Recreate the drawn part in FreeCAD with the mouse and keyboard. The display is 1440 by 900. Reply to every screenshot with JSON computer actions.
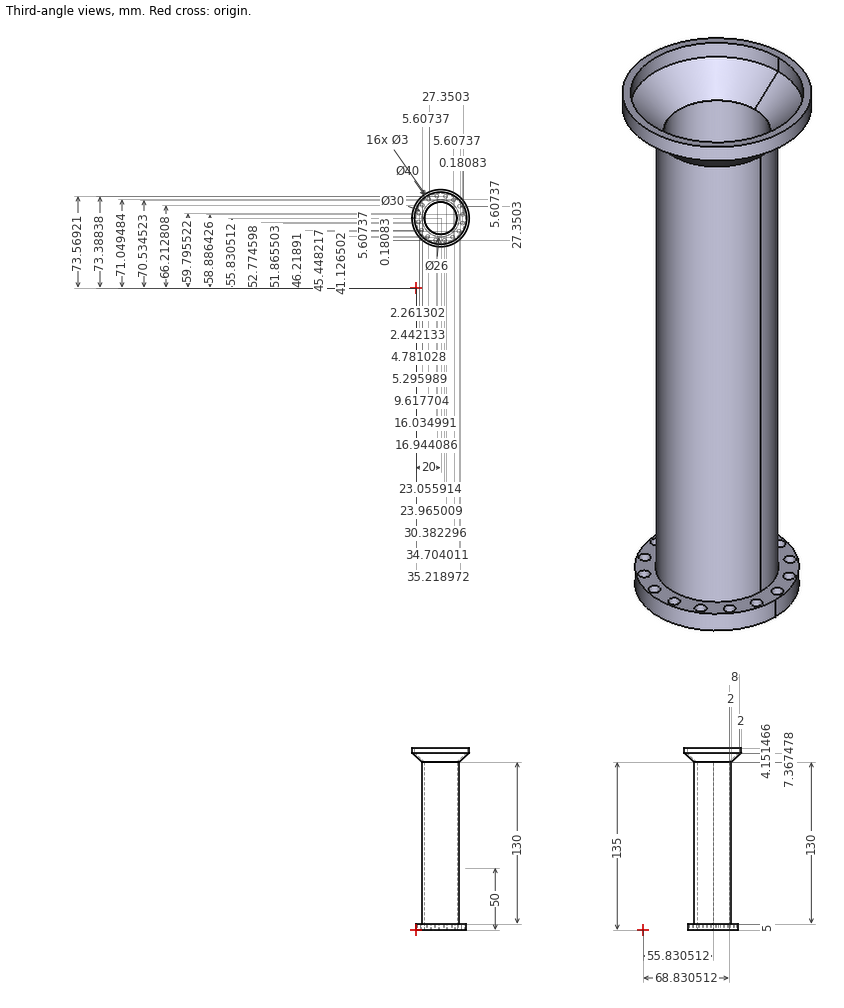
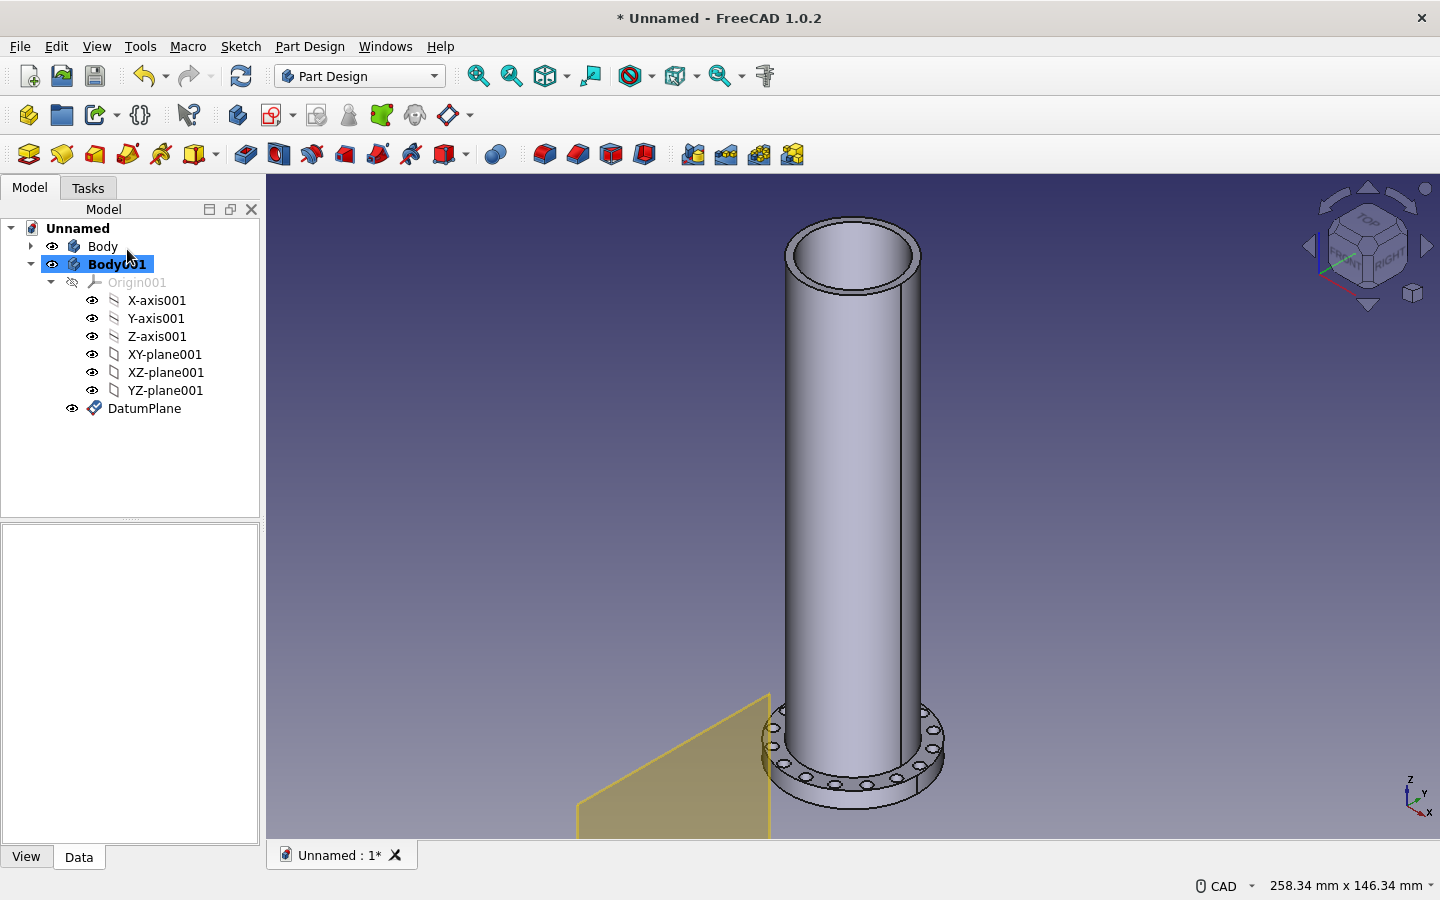
{"action": "left_click", "coordinate": [117, 408]}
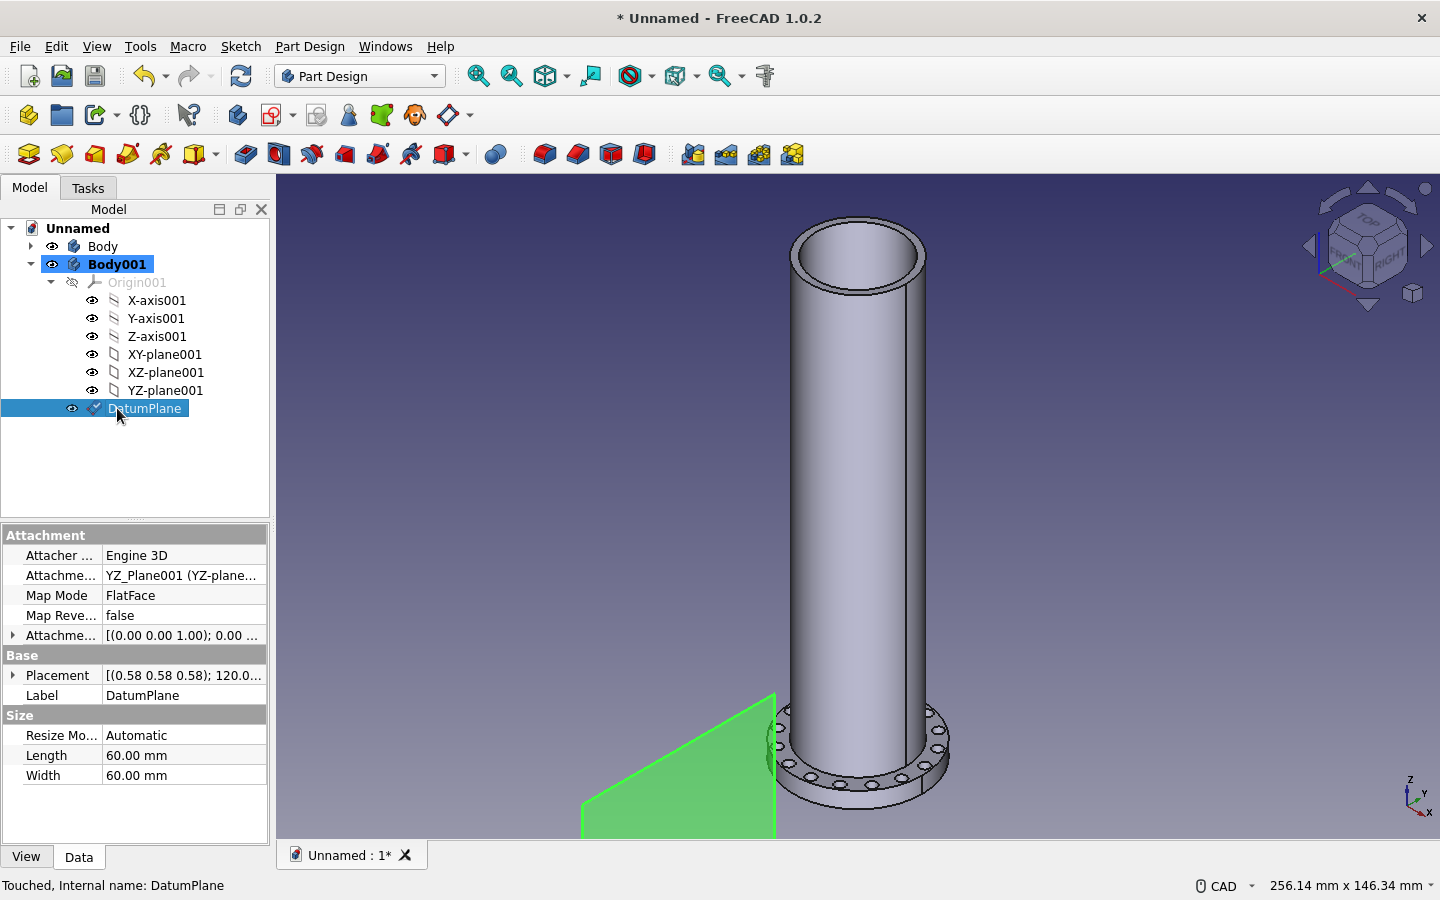
{"action": "left_click", "coordinate": [270, 116]}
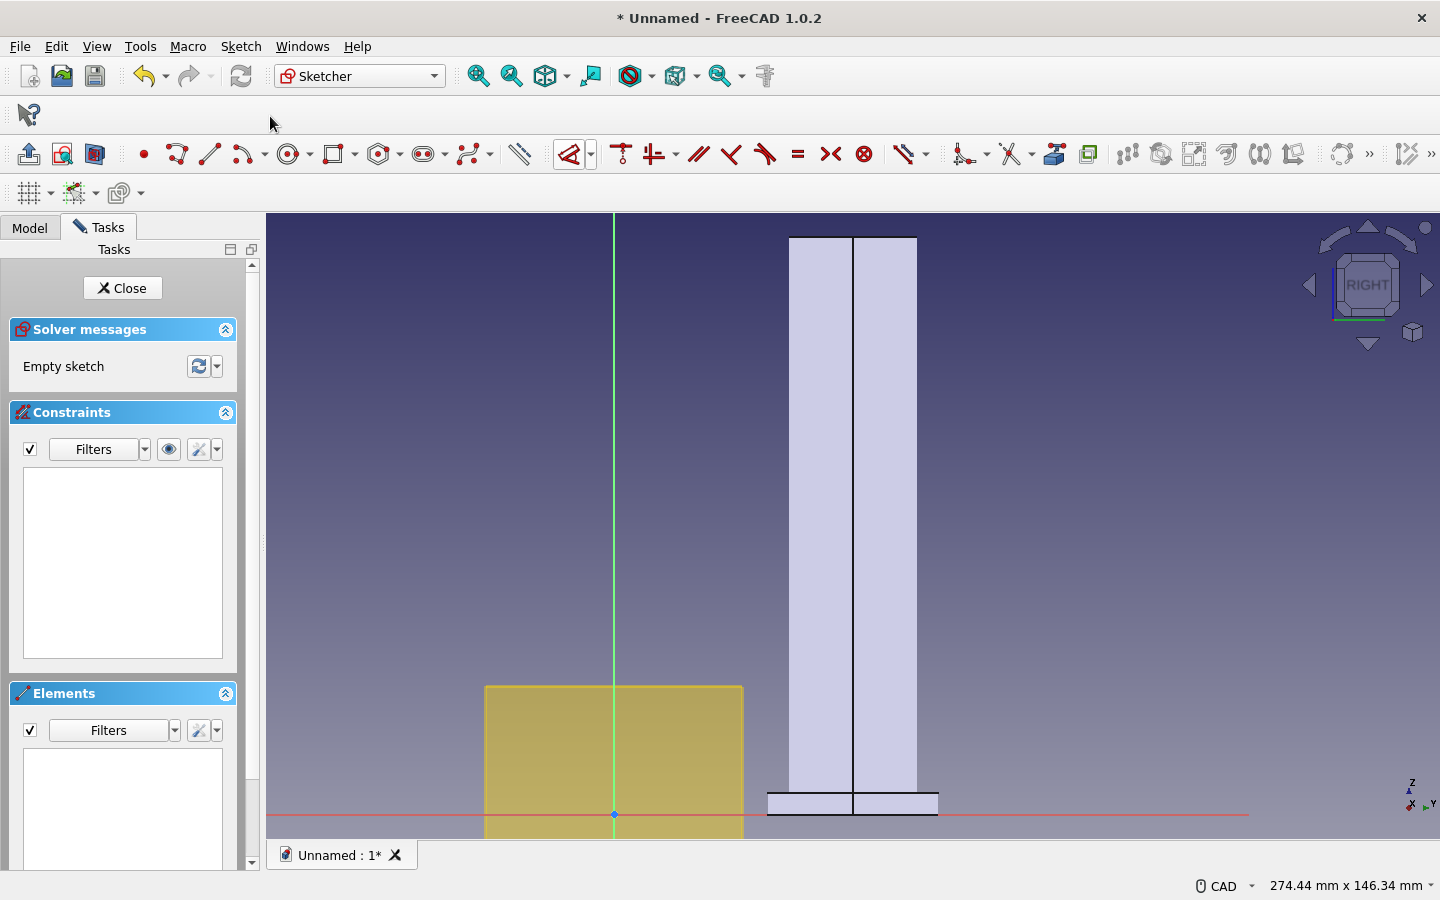
{"action": "scroll", "coordinate": [784, 526], "scroll_direction": "down", "scroll_amount": 5}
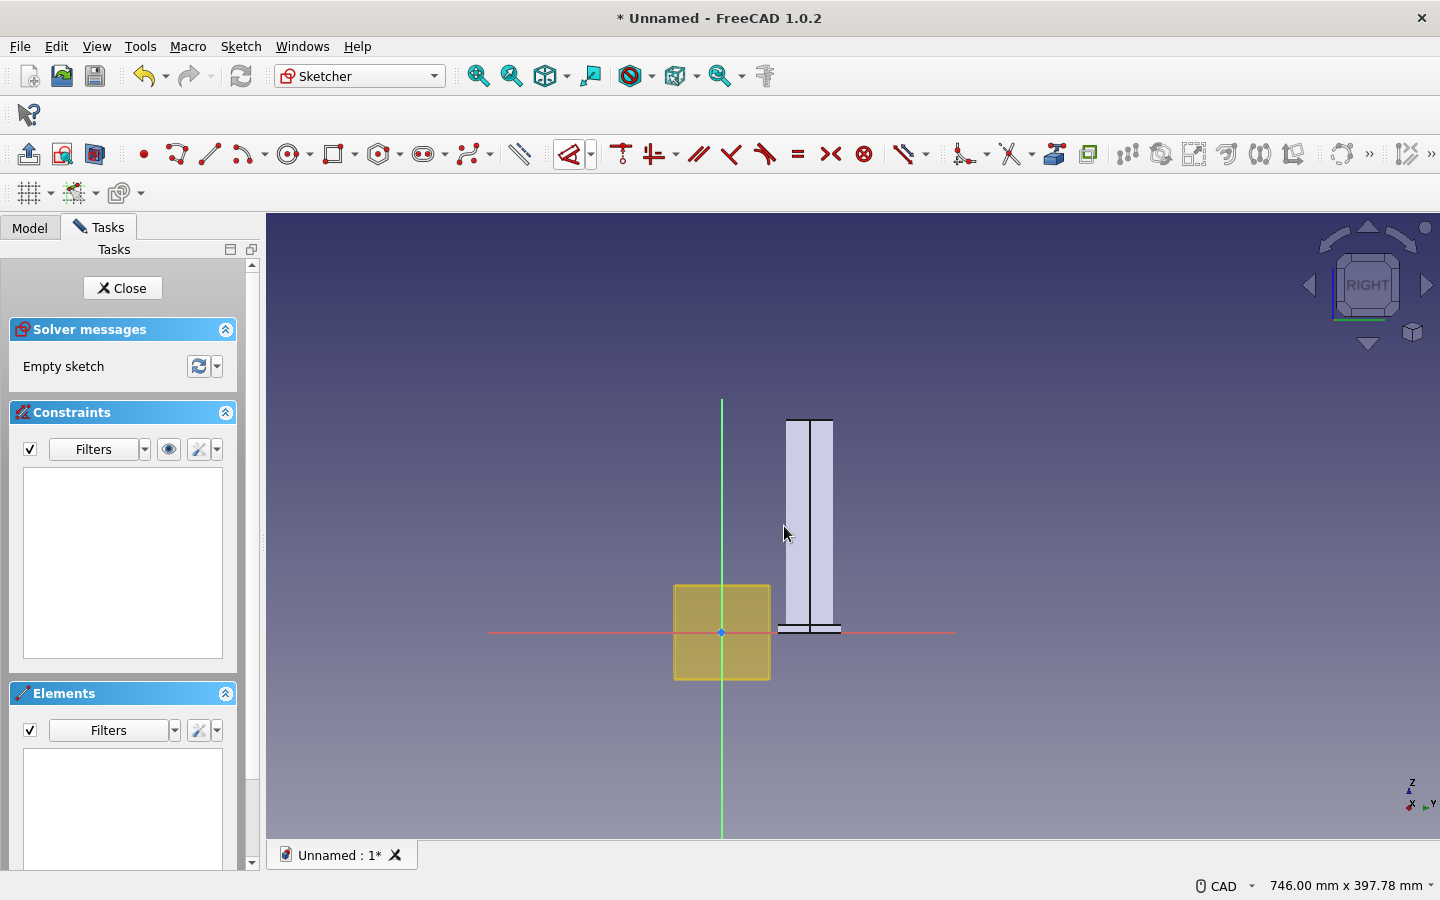
{"action": "scroll", "coordinate": [830, 405], "scroll_direction": "up", "scroll_amount": 15}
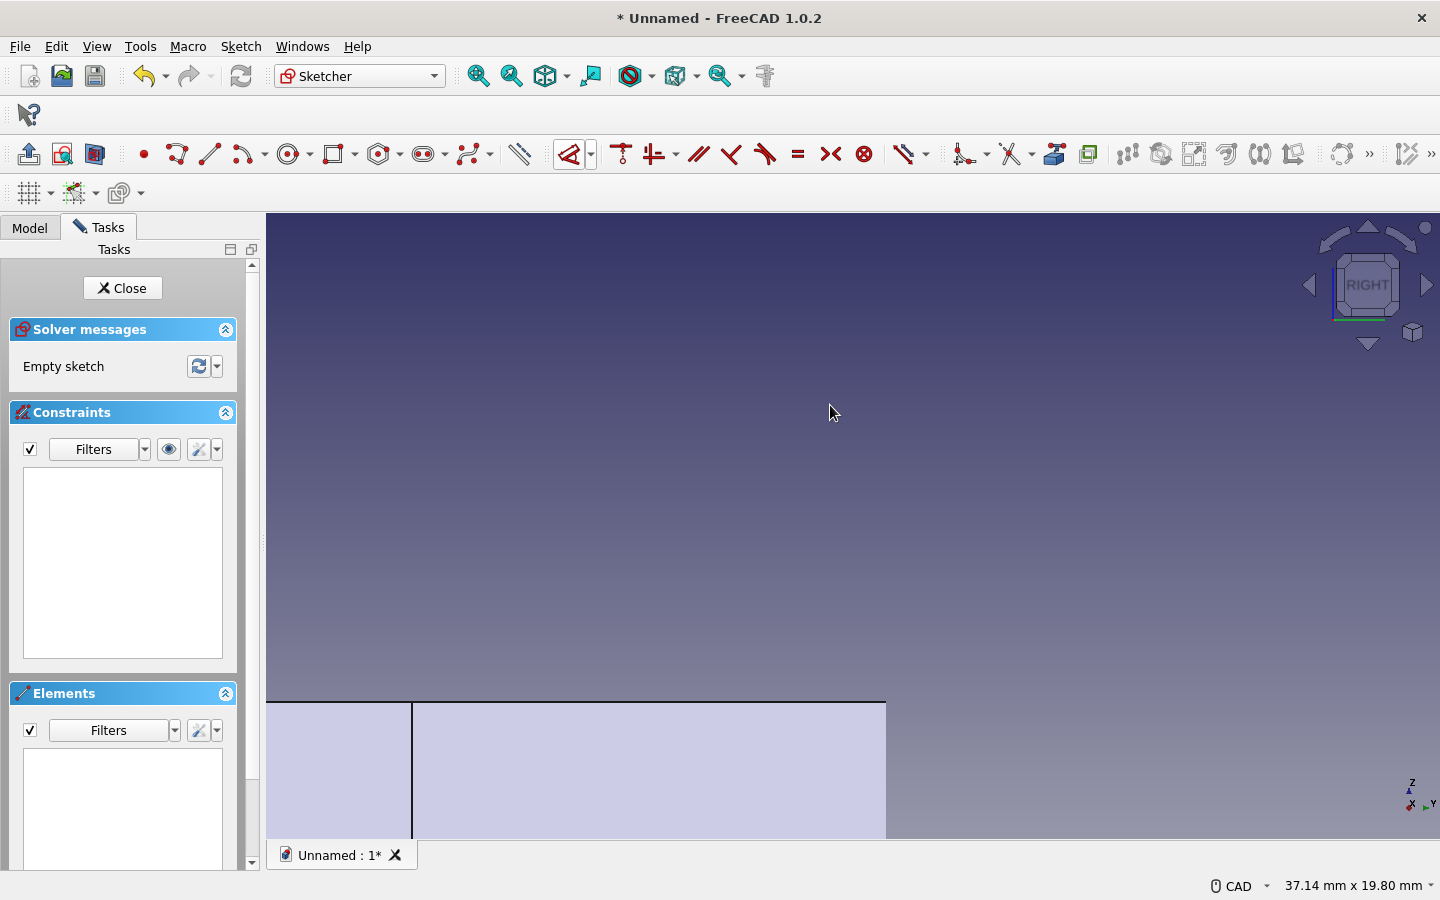
{"action": "left_click", "coordinate": [177, 154]}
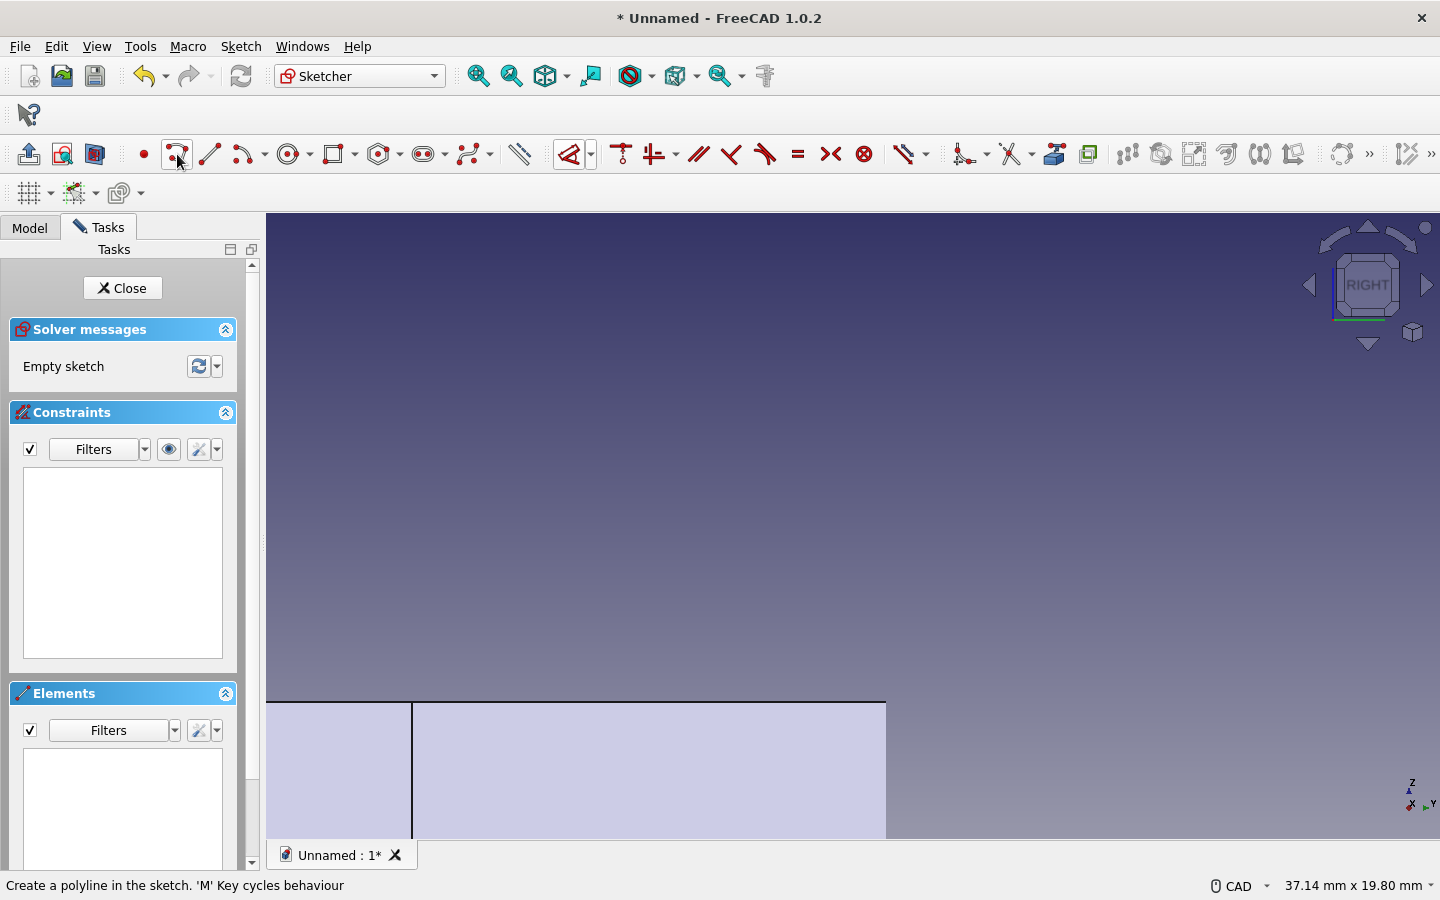
{"action": "left_click", "coordinate": [823, 702]}
{"action": "left_click", "coordinate": [1076, 469]}
{"action": "left_click", "coordinate": [1076, 338]}
{"action": "left_click", "coordinate": [1139, 338]}
{"action": "left_click", "coordinate": [1139, 469]}
{"action": "left_click", "coordinate": [886, 702]}
{"action": "left_click", "coordinate": [823, 703]}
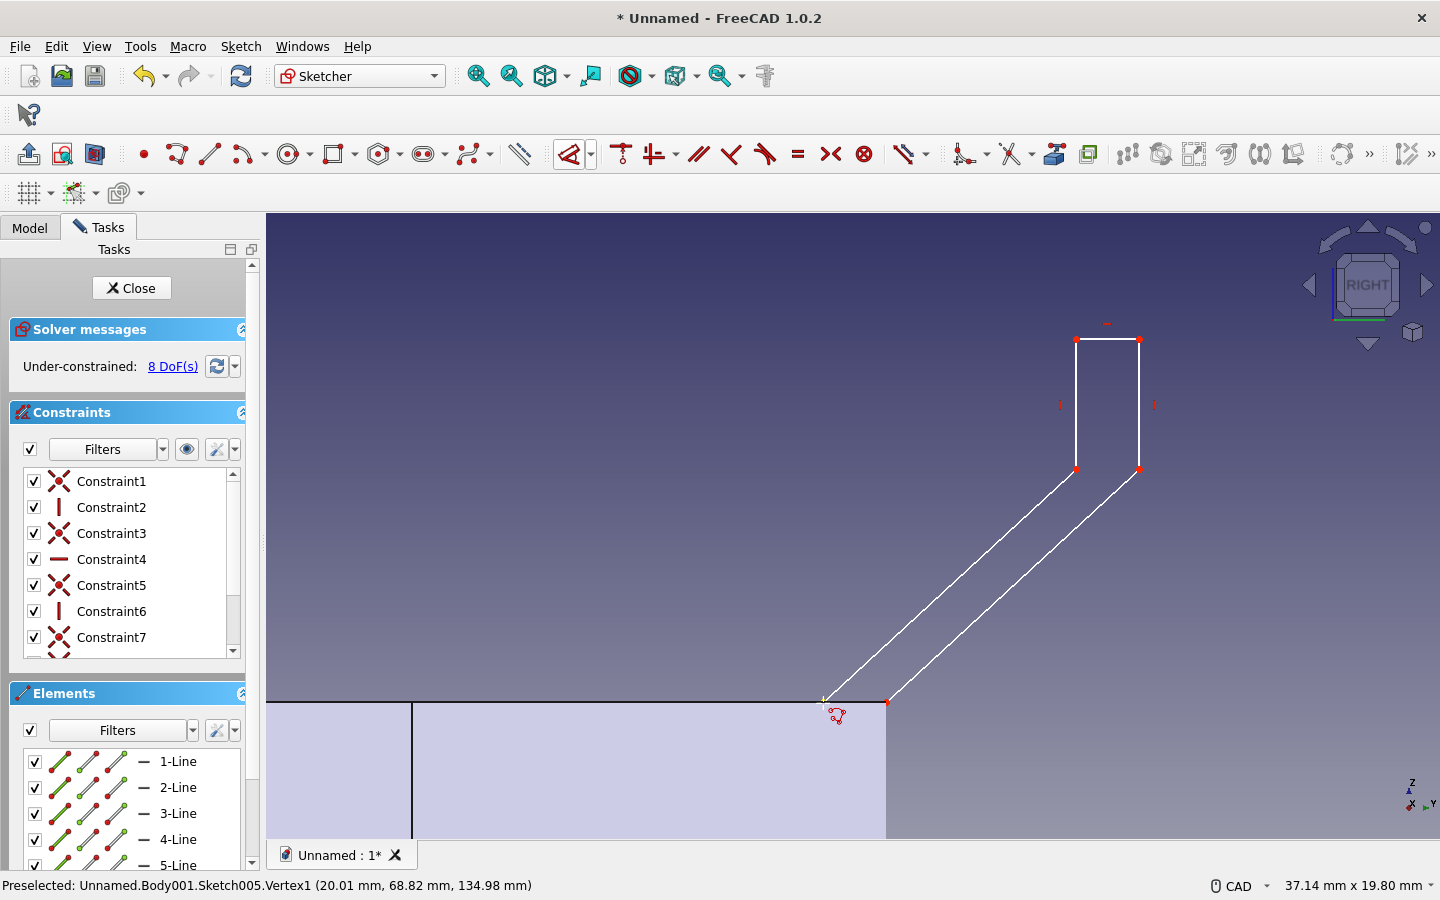
{"action": "key", "text": "g l"}